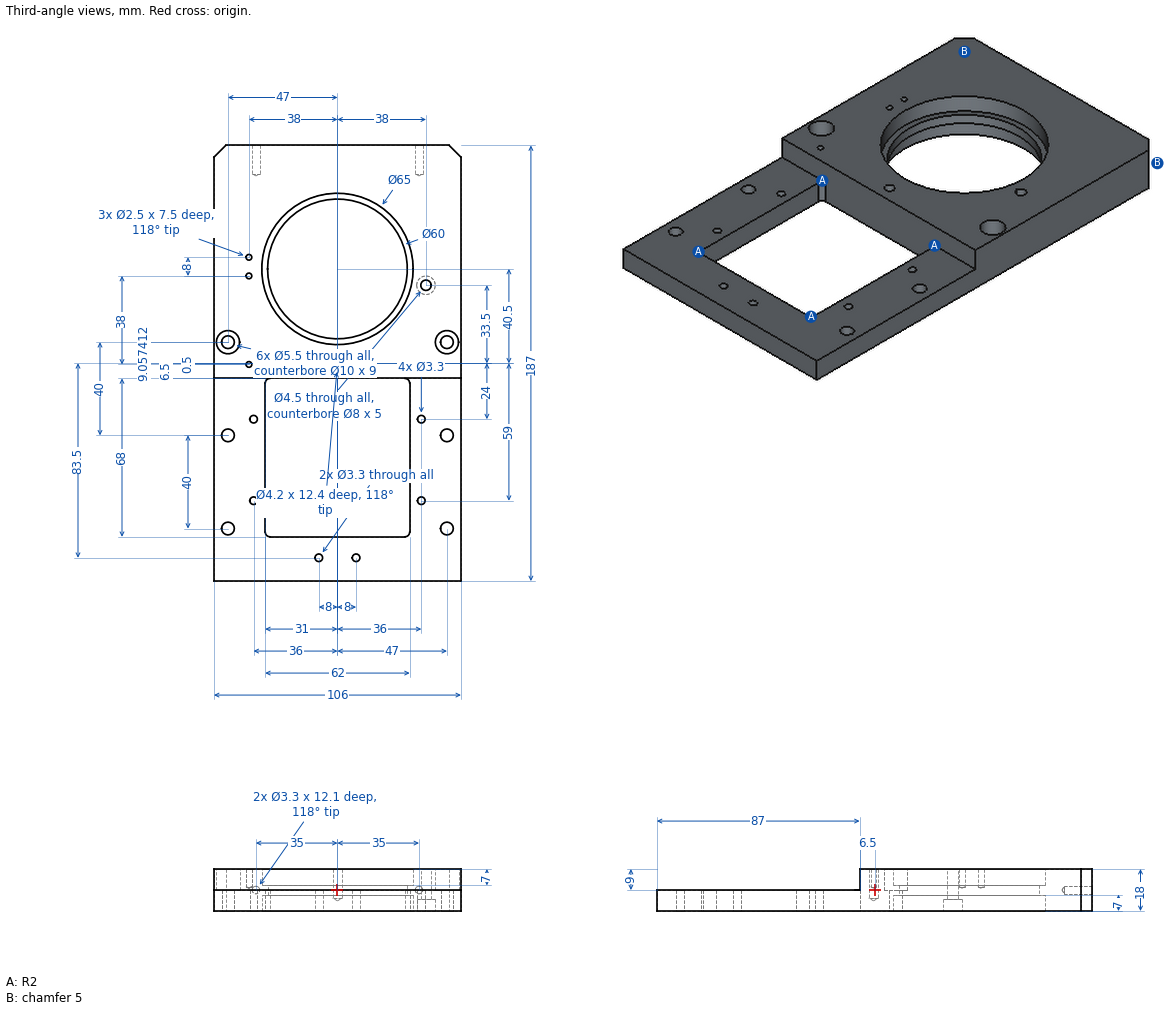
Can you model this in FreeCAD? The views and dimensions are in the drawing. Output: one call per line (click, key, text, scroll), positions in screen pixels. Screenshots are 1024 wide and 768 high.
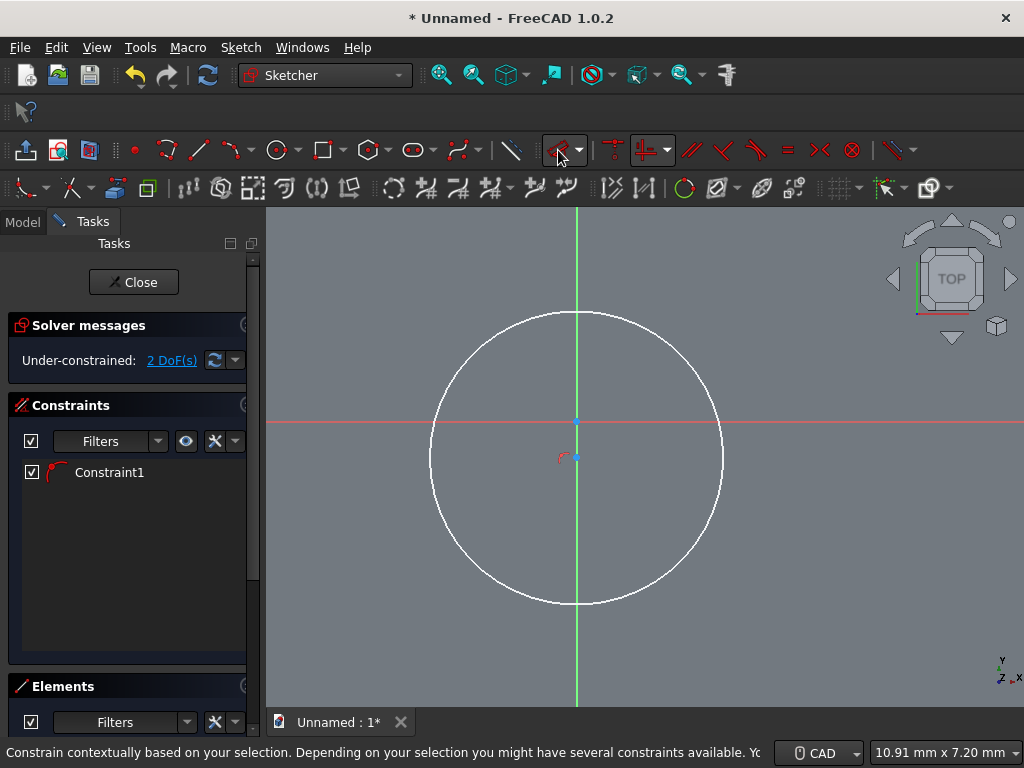
click(680, 354)
click(703, 331)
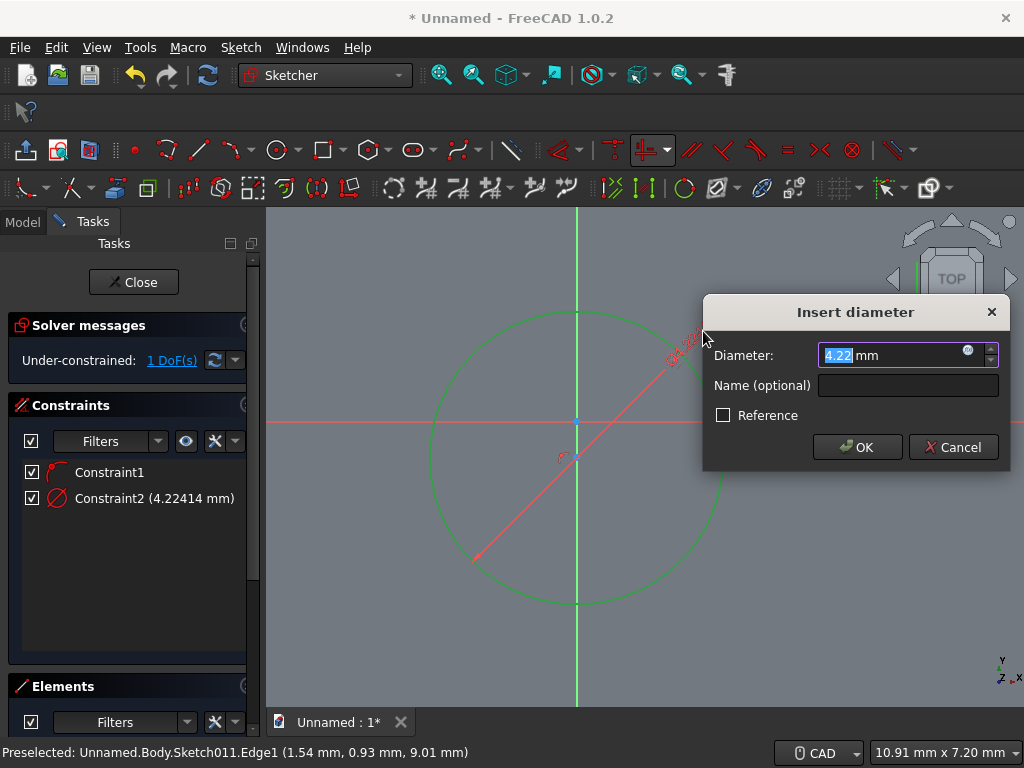
text(4.2)
key(Return)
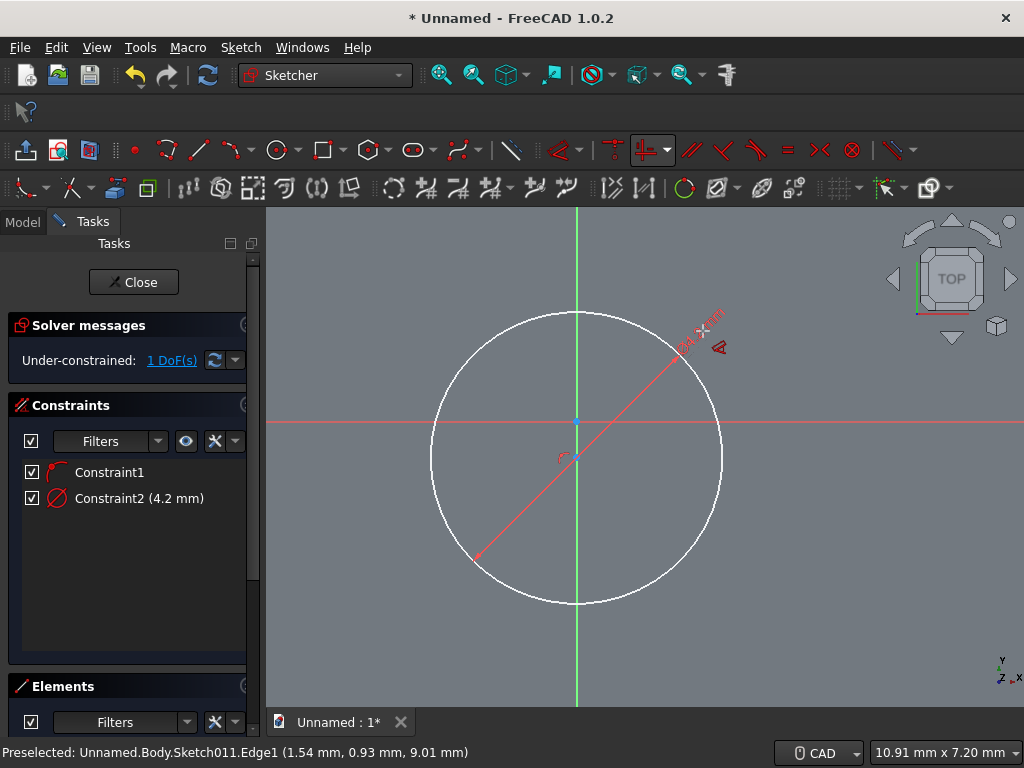
click(577, 458)
click(611, 440)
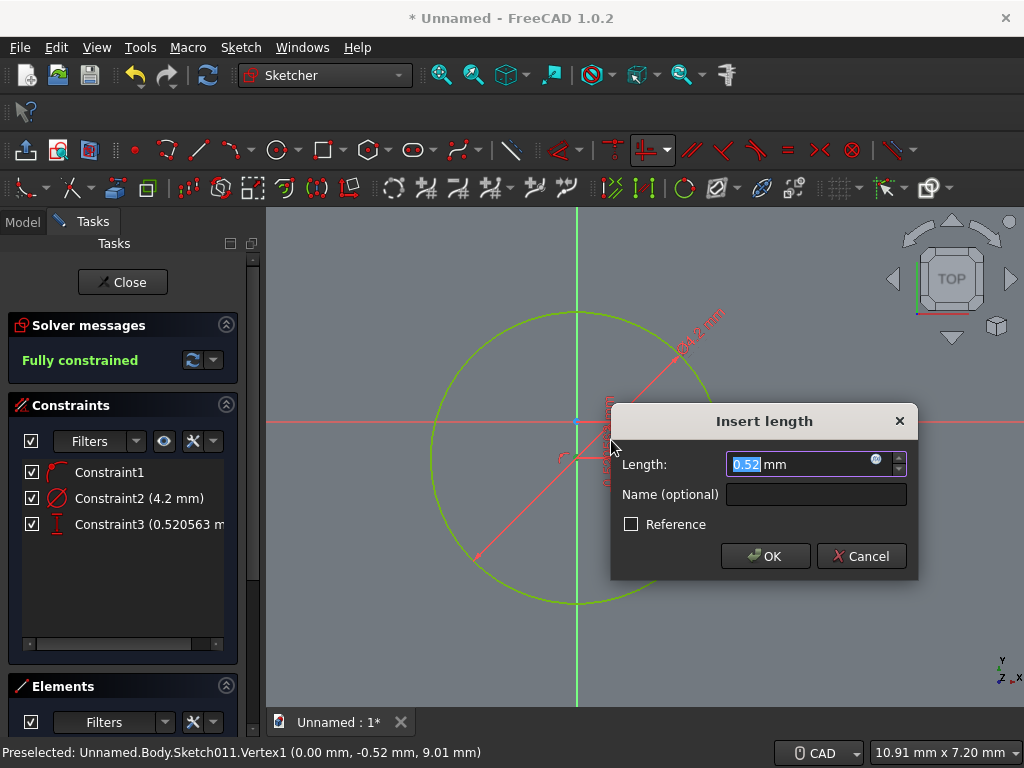
text(0.5)
key(Return)
key(Escape)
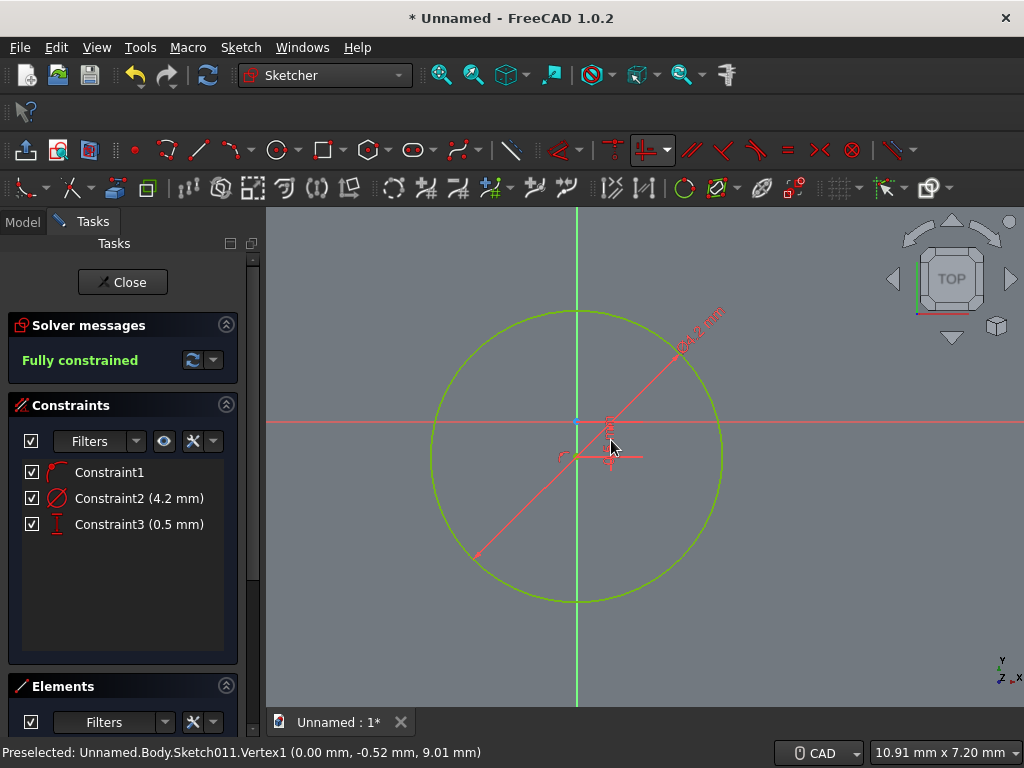
click(123, 282)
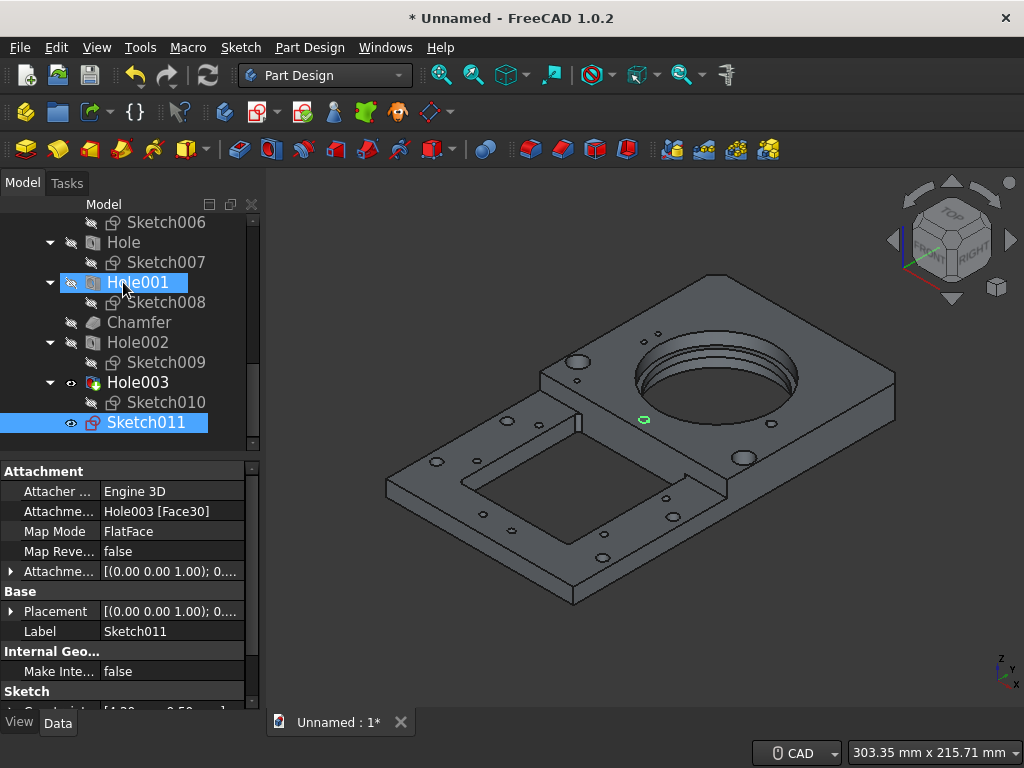
click(272, 150)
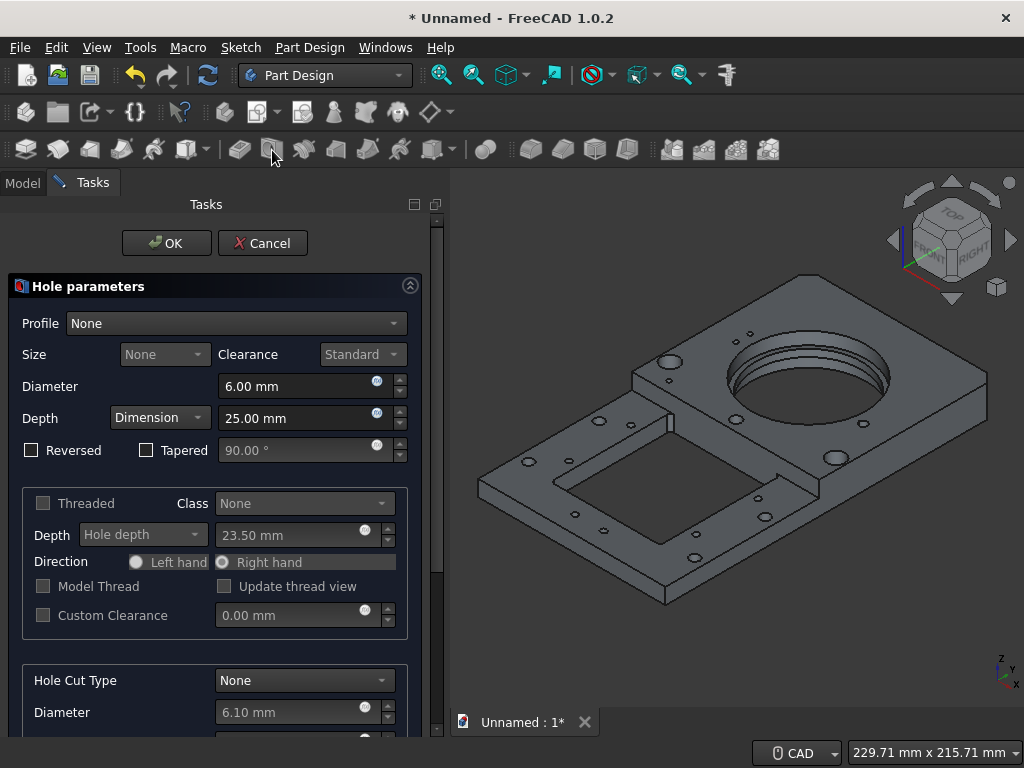
triple_click(305, 386)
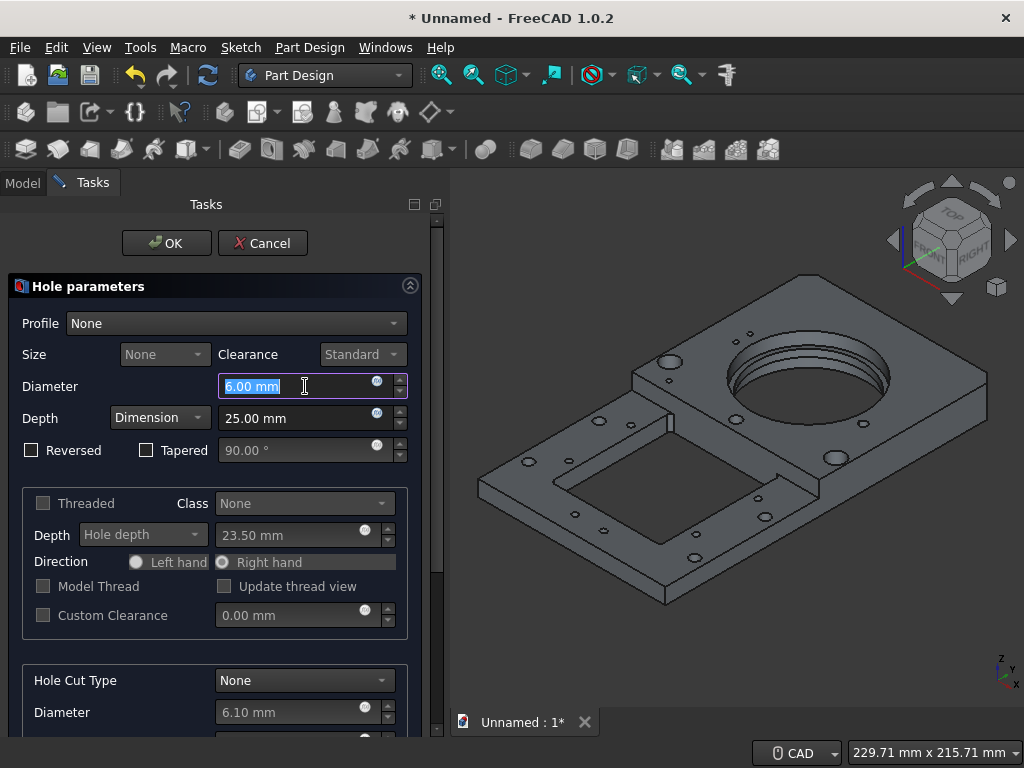
text(4.2)
key(Tab)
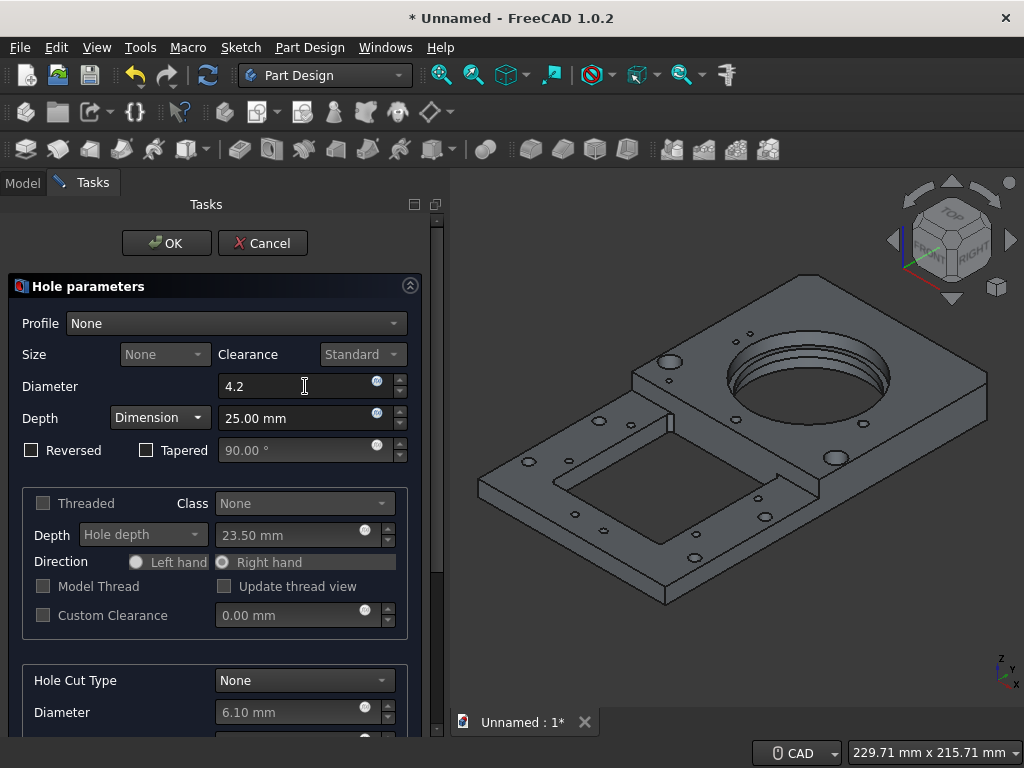
triple_click(305, 418)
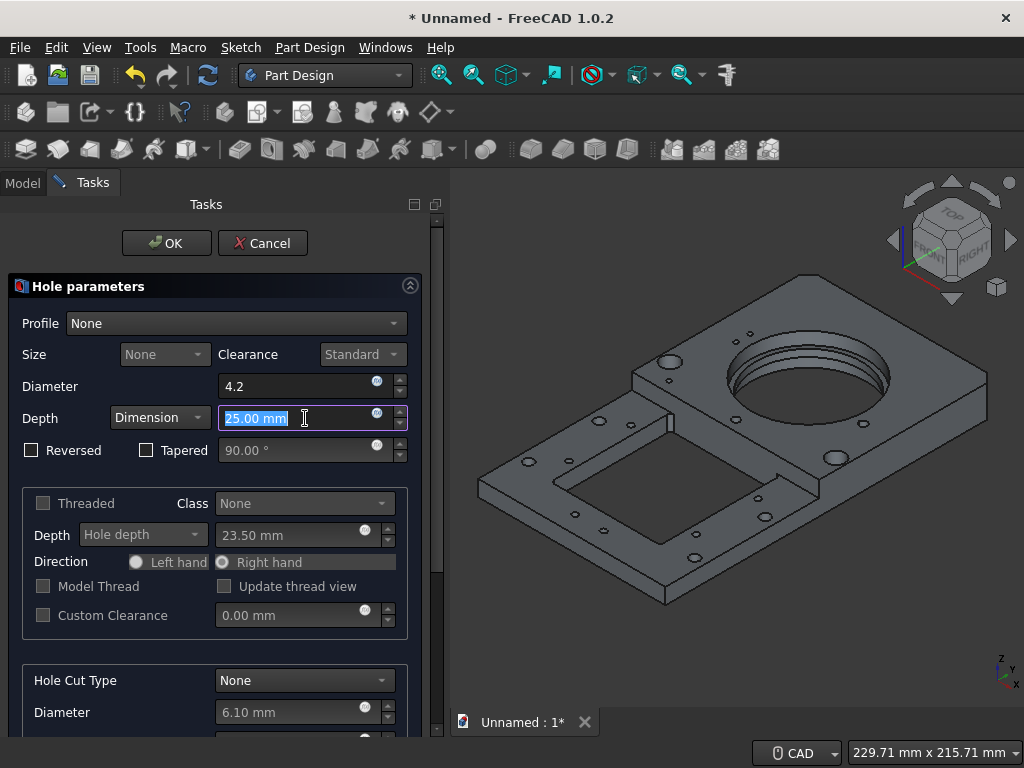
text(12.4)
key(Tab)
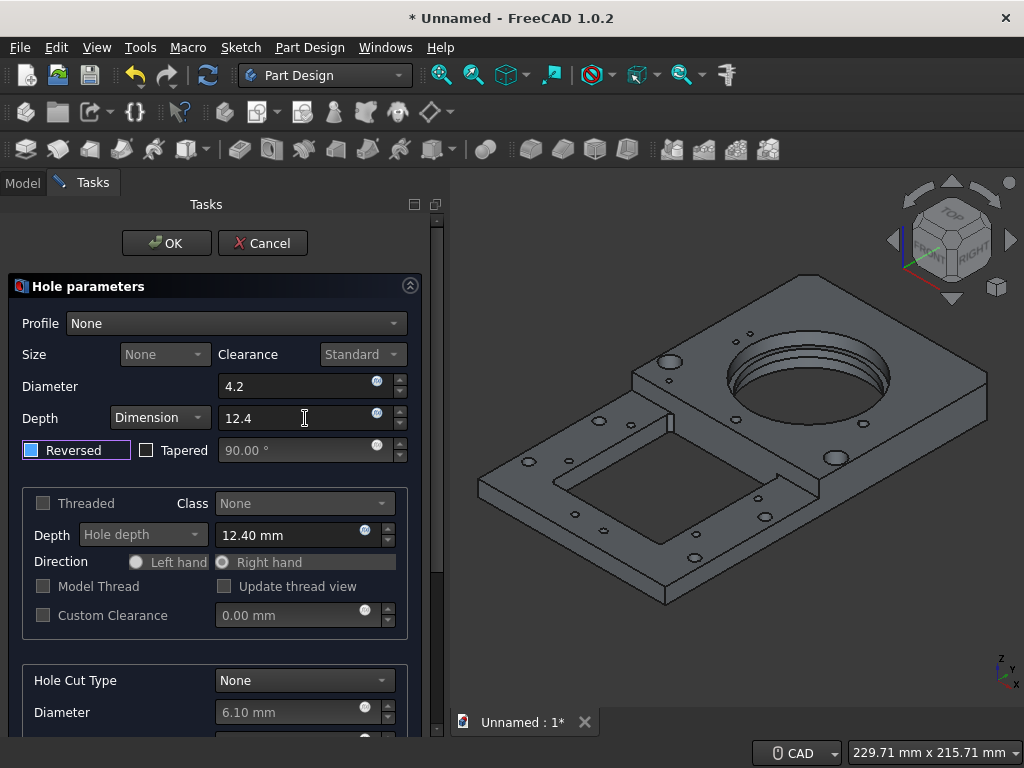
click(167, 243)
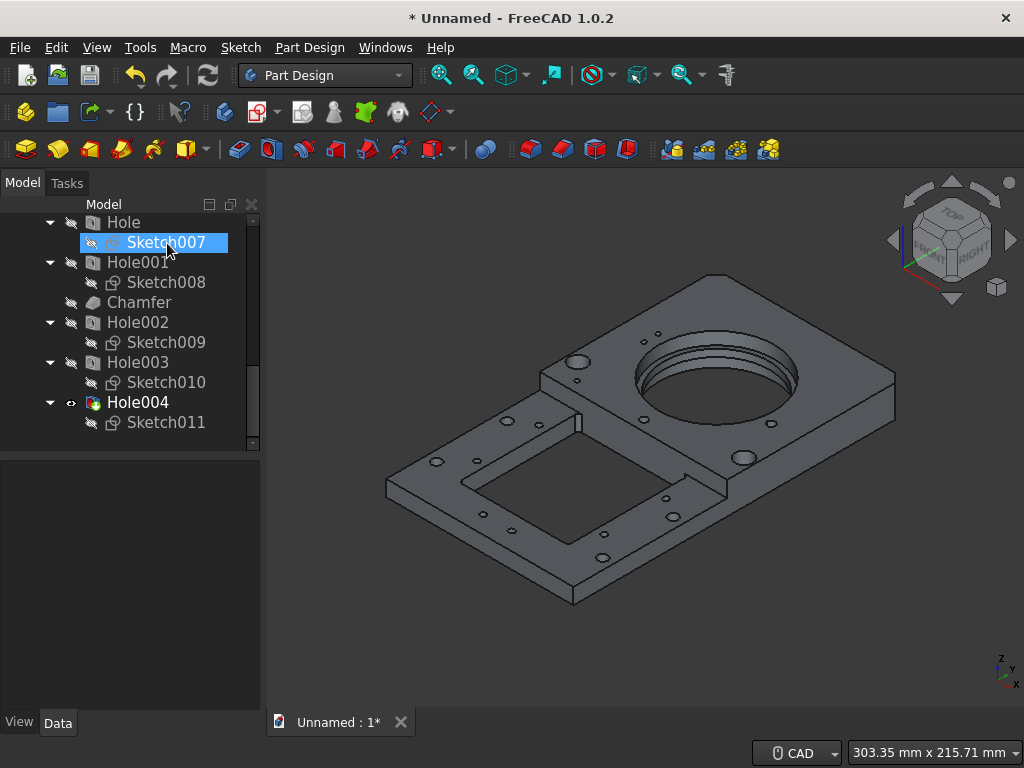
key(4)